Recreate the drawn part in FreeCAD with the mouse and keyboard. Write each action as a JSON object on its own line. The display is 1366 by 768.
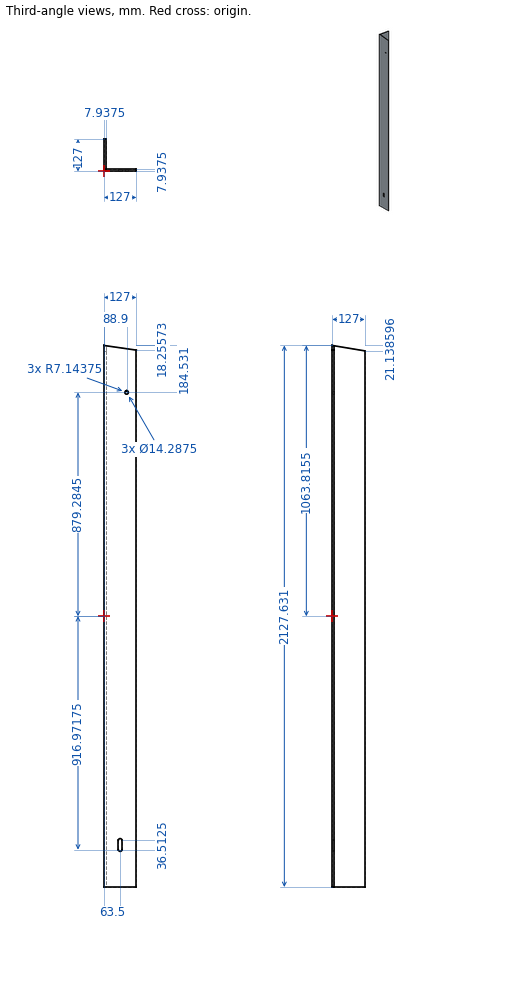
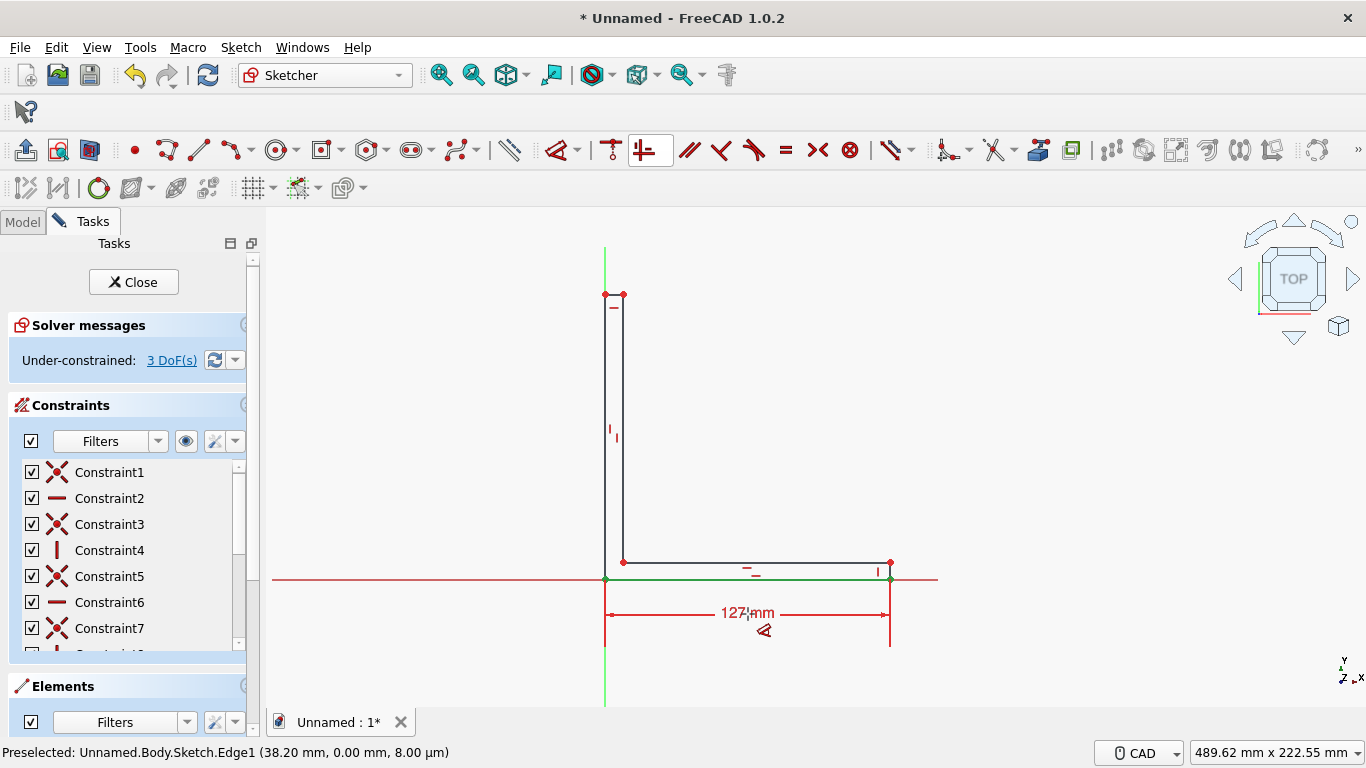
{"action": "left_click", "coordinate": [605, 380]}
{"action": "left_click", "coordinate": [571, 437]}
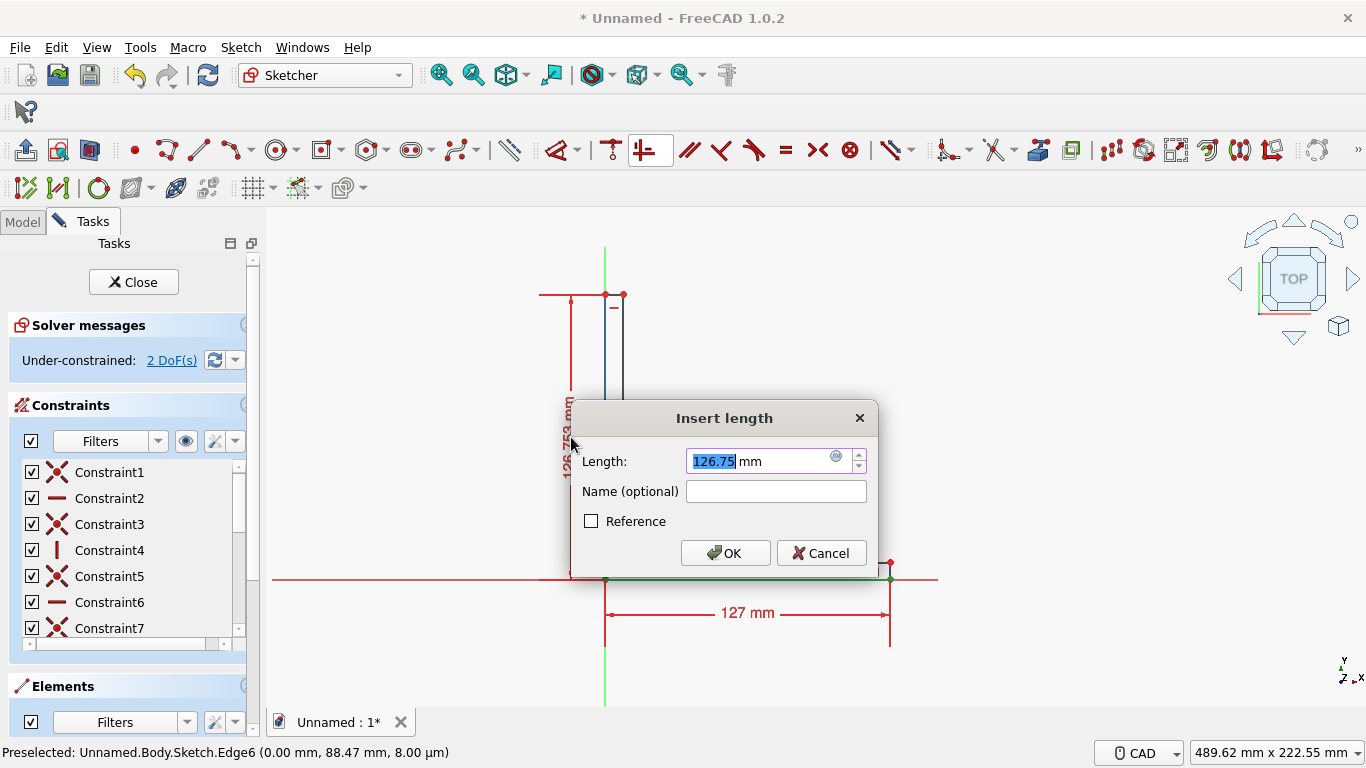
{"action": "type", "text": "127"}
{"action": "key", "text": "Return"}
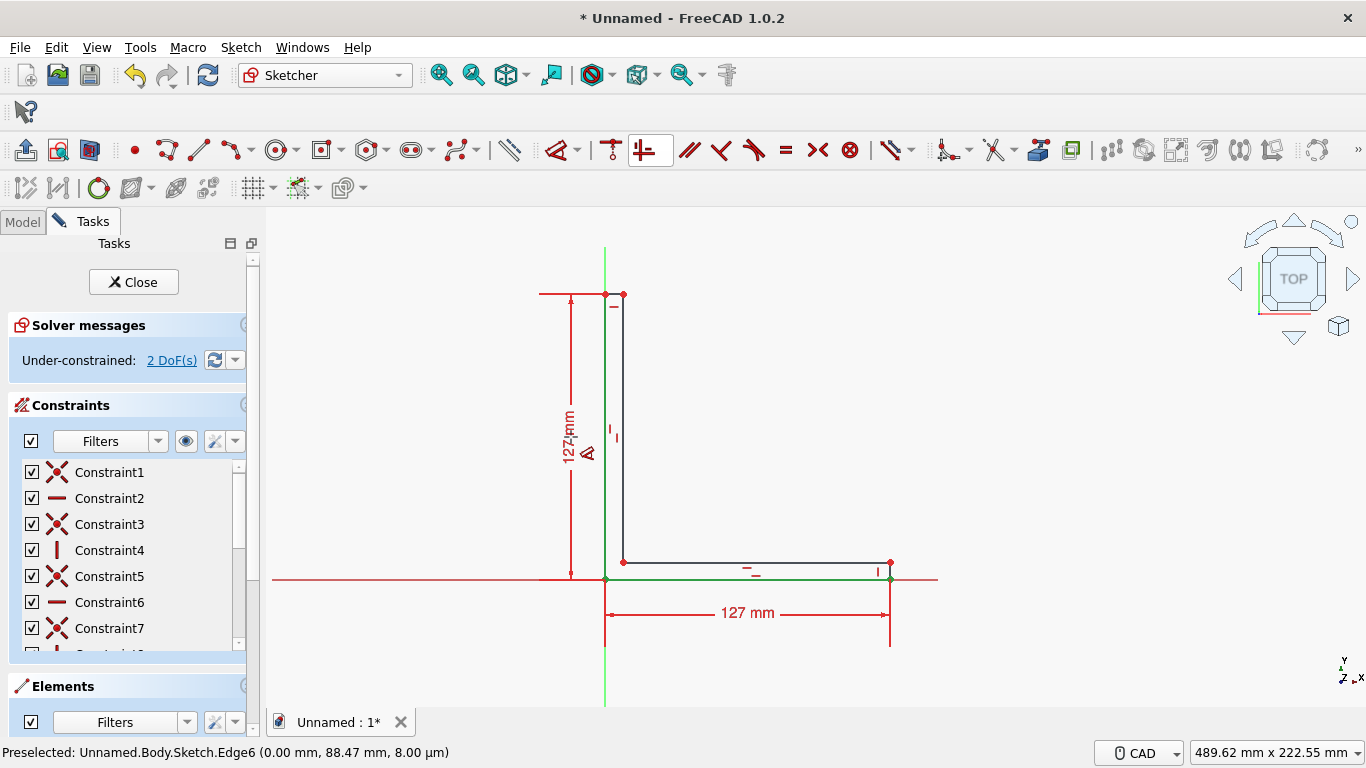
{"action": "scroll", "coordinate": [891, 571], "scroll_direction": "up", "scroll_amount": 5}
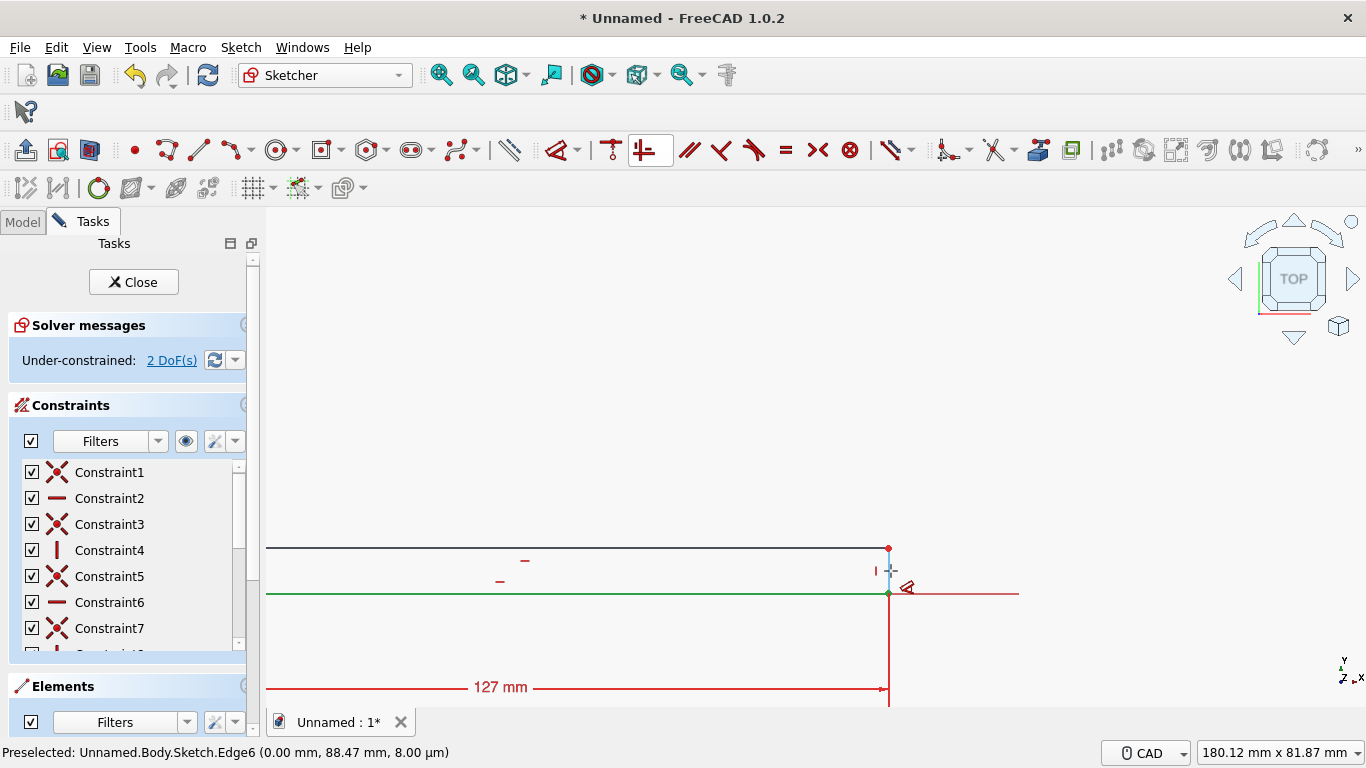
{"action": "left_click", "coordinate": [889, 571]}
{"action": "left_click", "coordinate": [923, 571]}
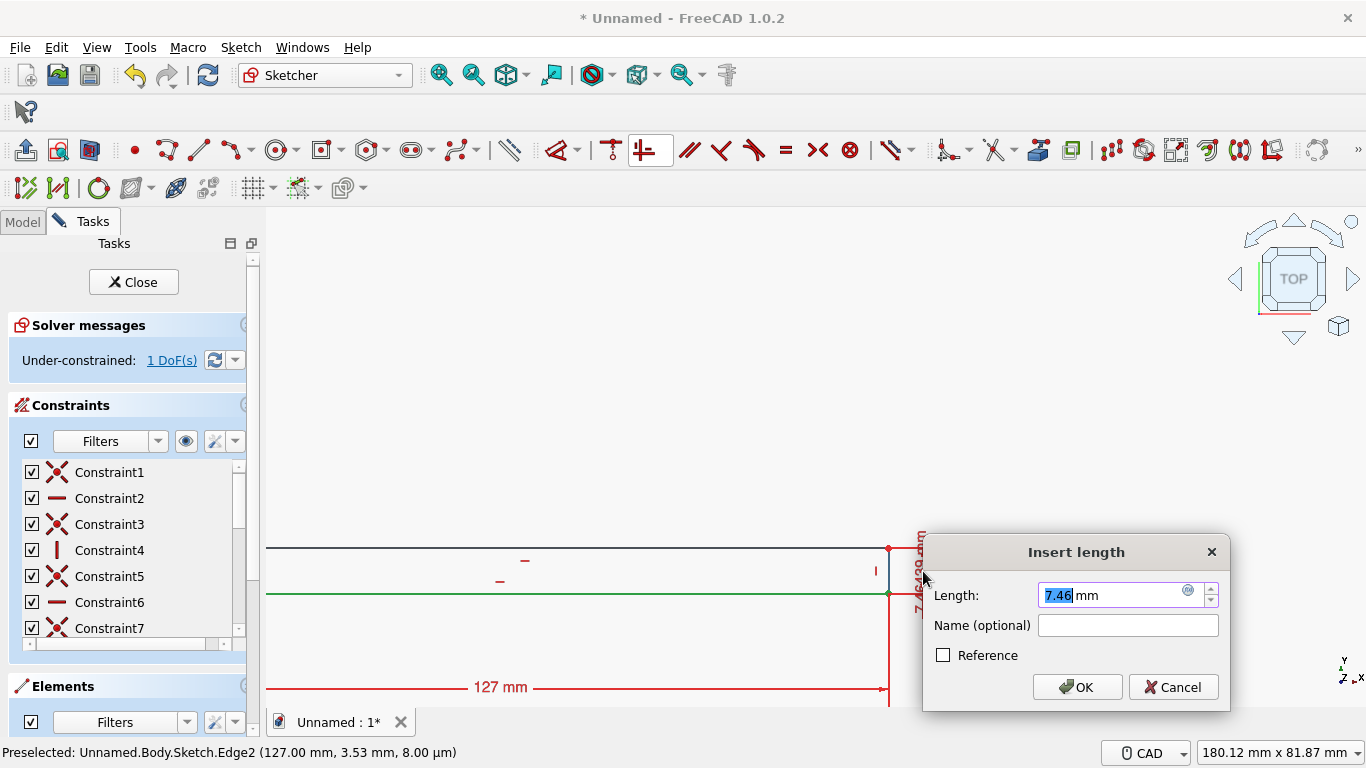
{"action": "type", "text": "7.9375"}
{"action": "key", "text": "Return"}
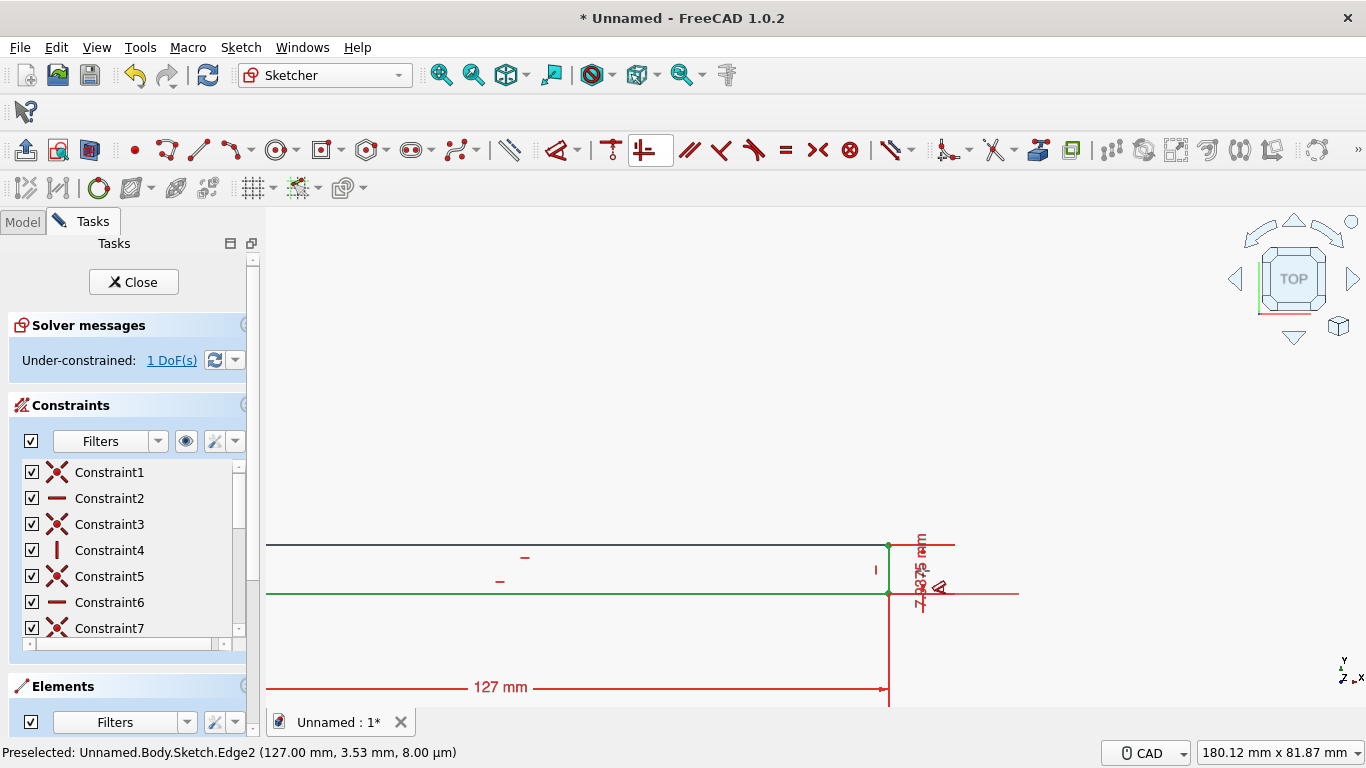
{"action": "scroll", "coordinate": [891, 603], "scroll_direction": "down", "scroll_amount": 5}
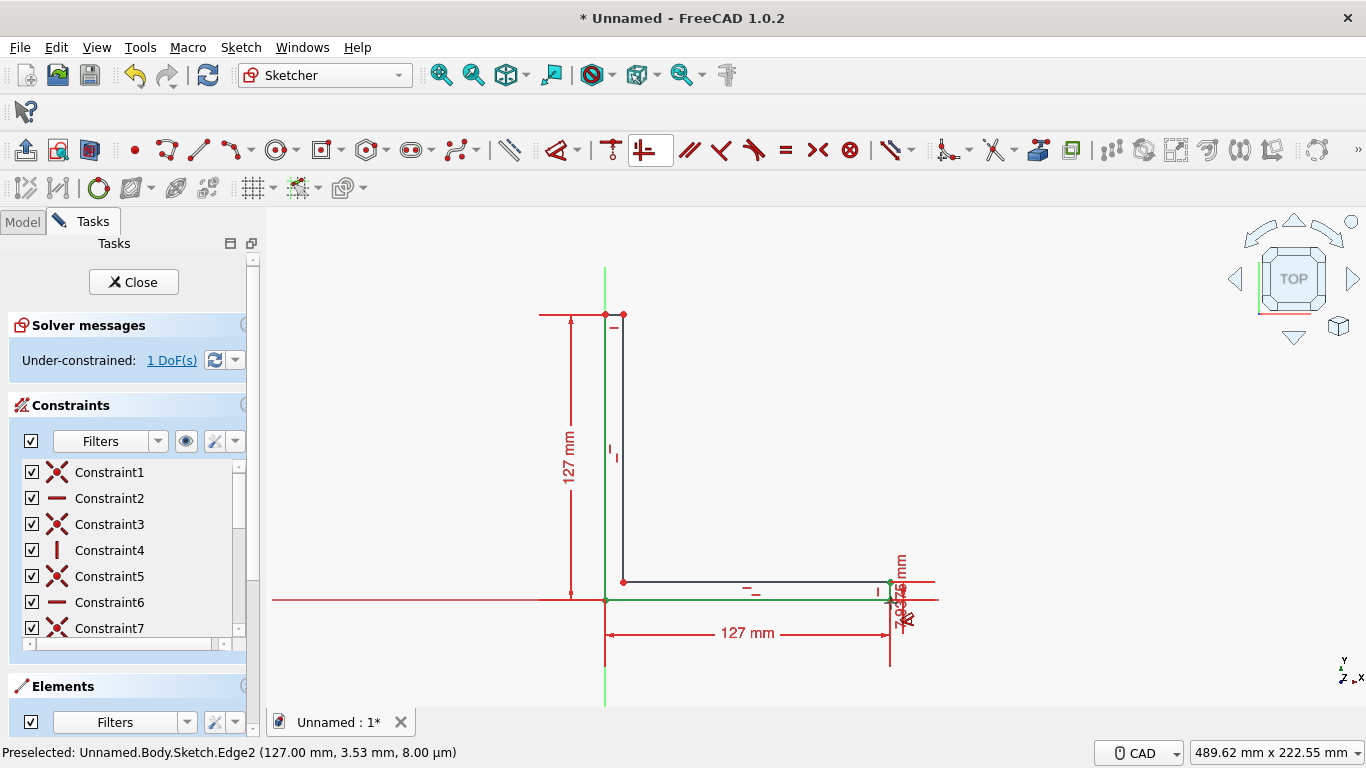
{"action": "scroll", "coordinate": [618, 315], "scroll_direction": "up", "scroll_amount": 5}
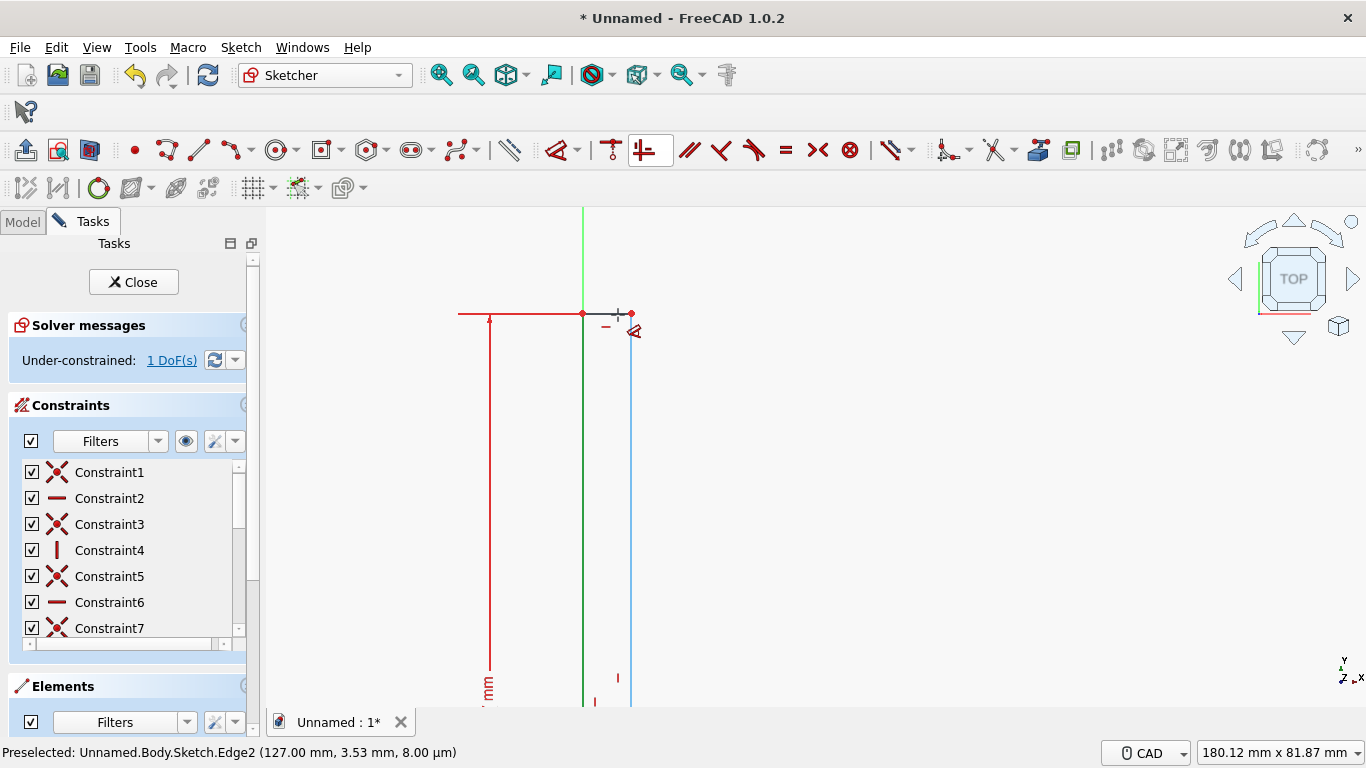
{"action": "left_click", "coordinate": [617, 314]}
{"action": "left_click", "coordinate": [607, 280]}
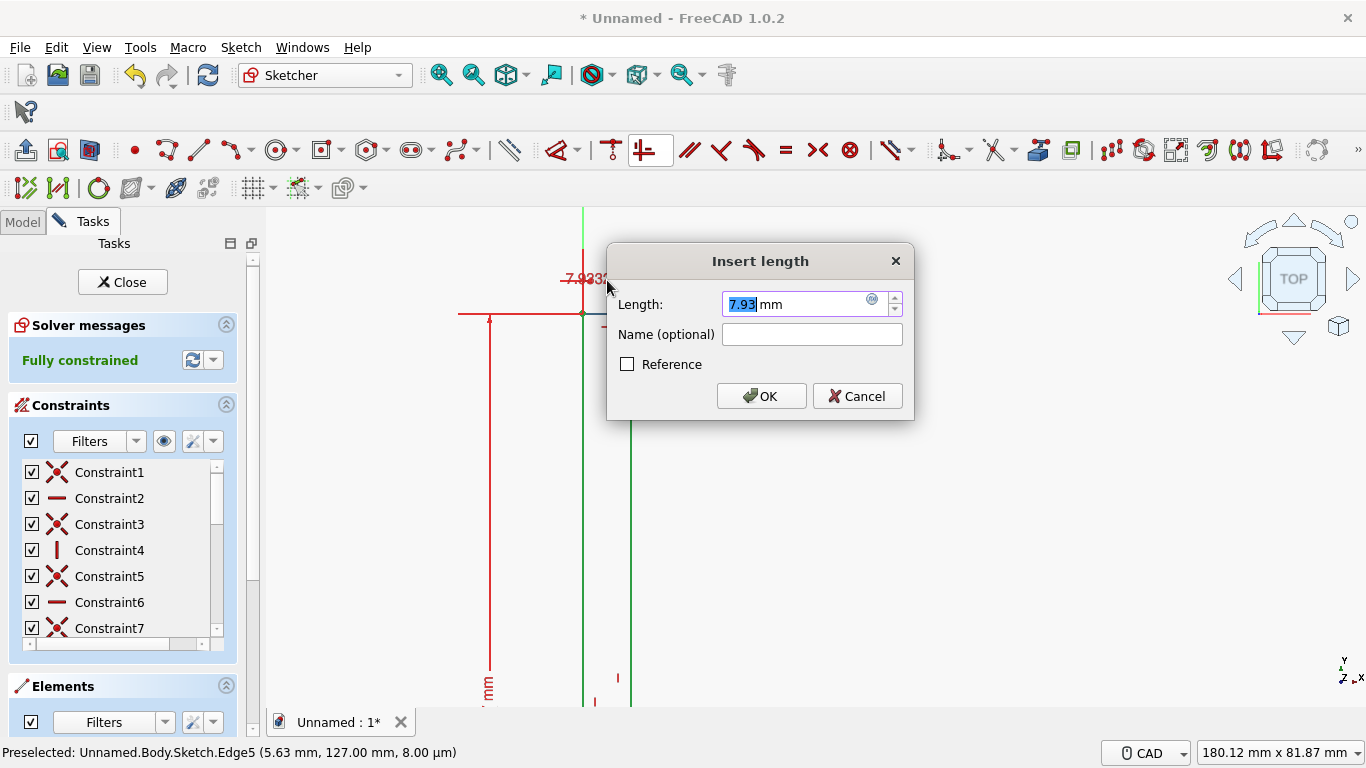
{"action": "type", "text": "7.9375"}
{"action": "key", "text": "Return"}
{"action": "key", "text": "Escape"}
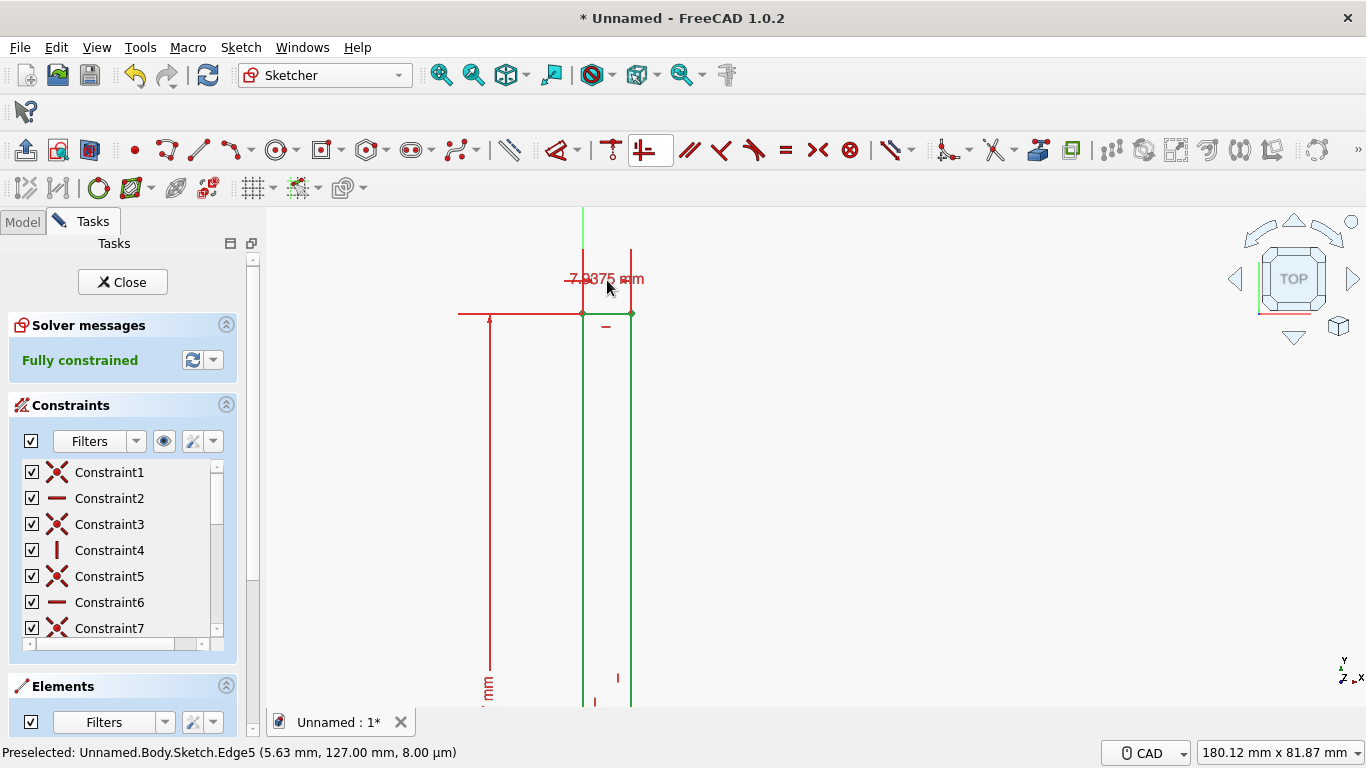
{"action": "left_click", "coordinate": [123, 282]}